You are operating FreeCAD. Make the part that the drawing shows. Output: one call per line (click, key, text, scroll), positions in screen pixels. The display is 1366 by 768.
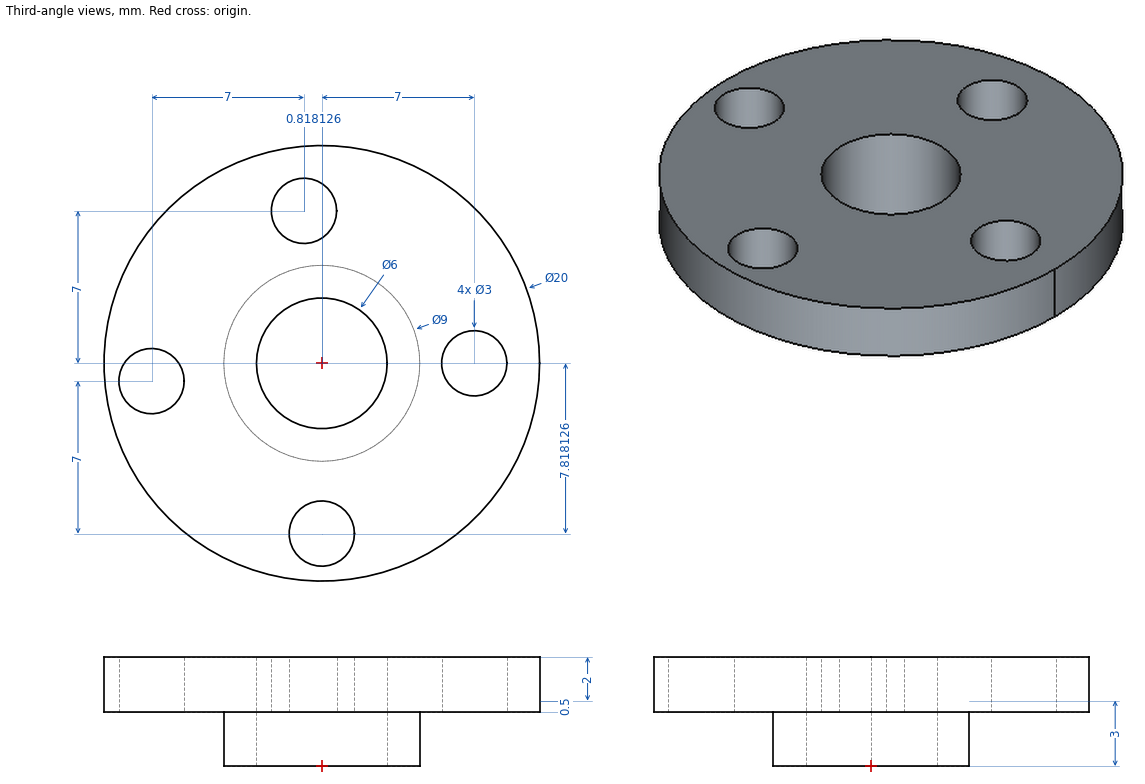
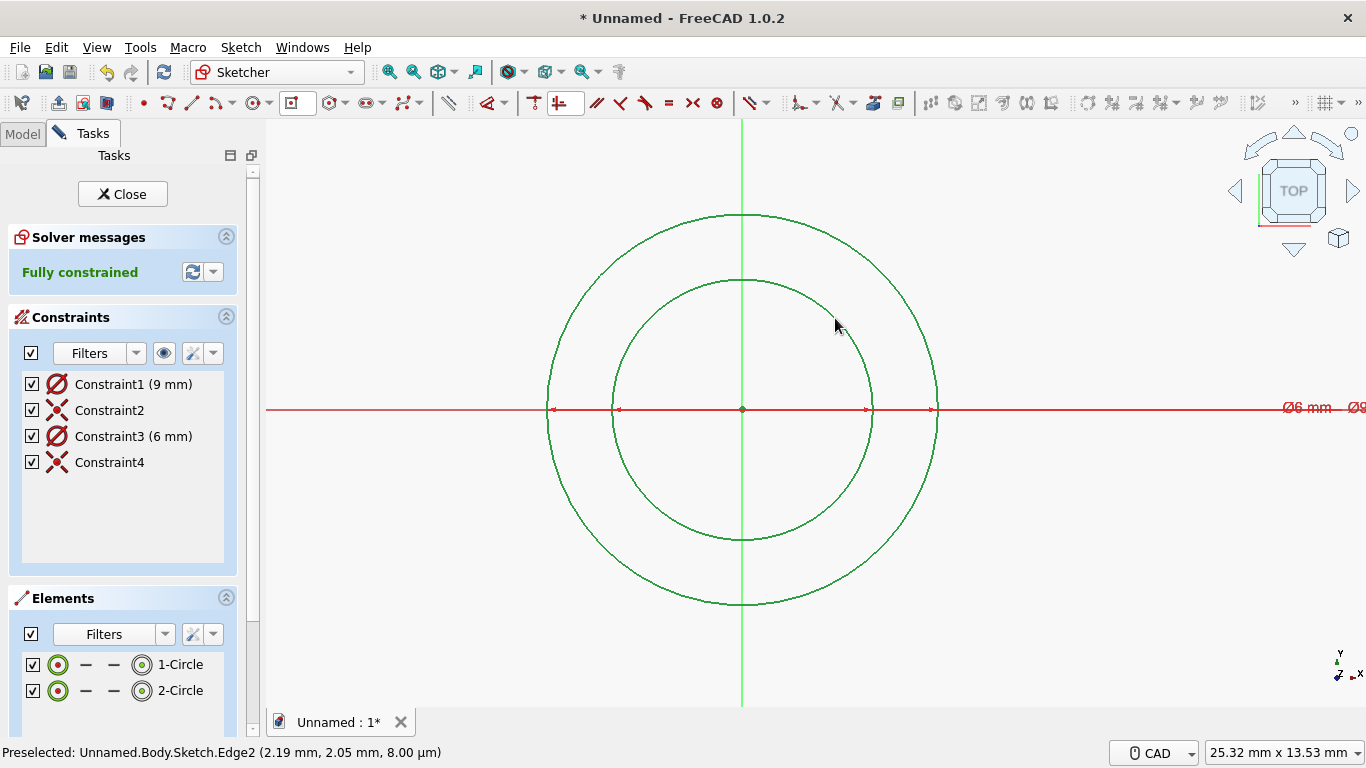
click(123, 194)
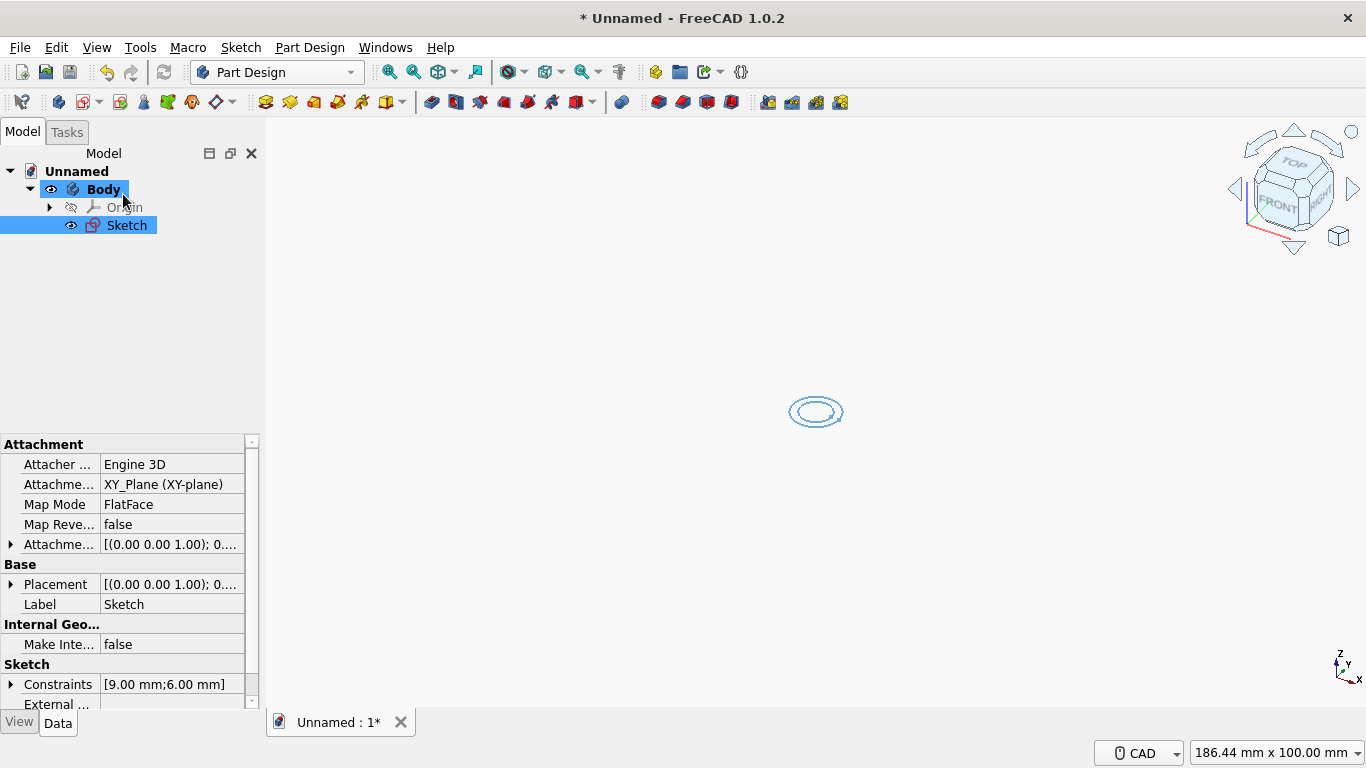
click(266, 102)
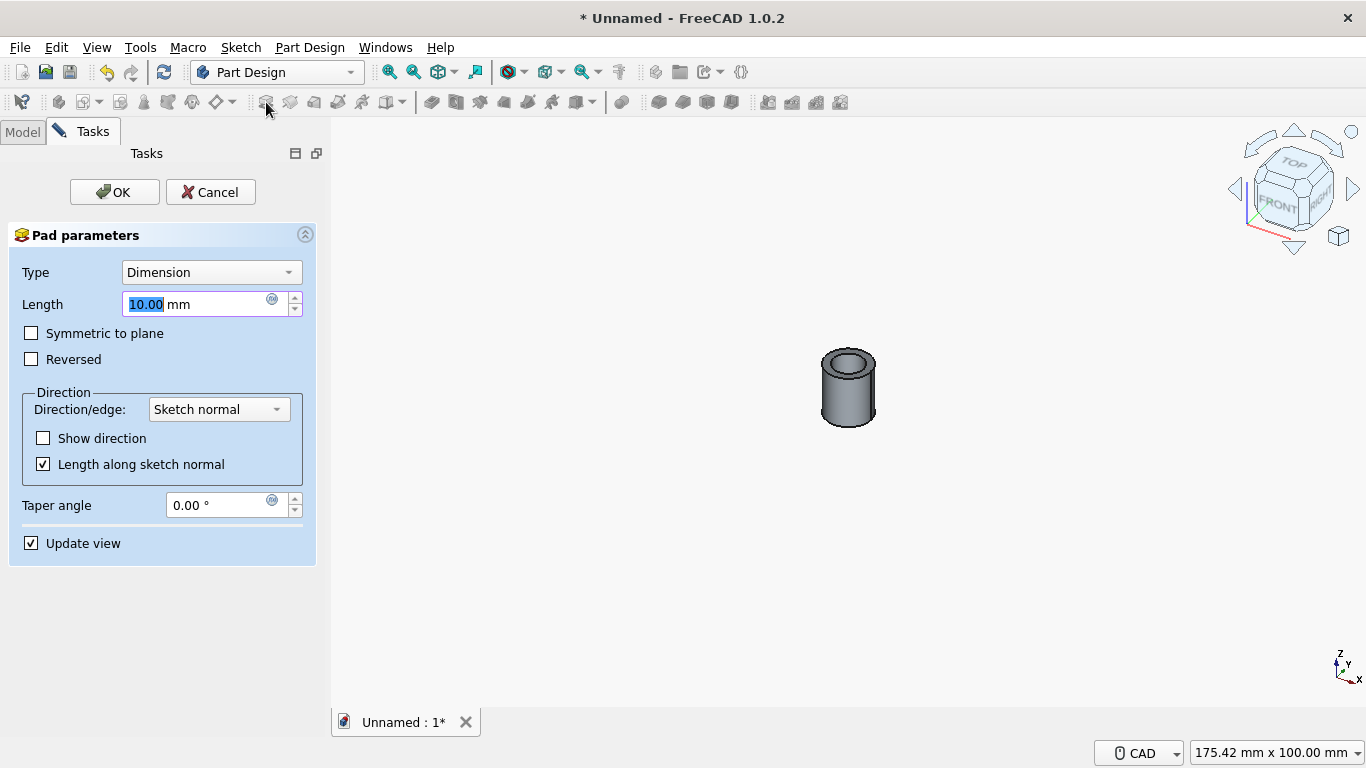
text(3)
key(Tab)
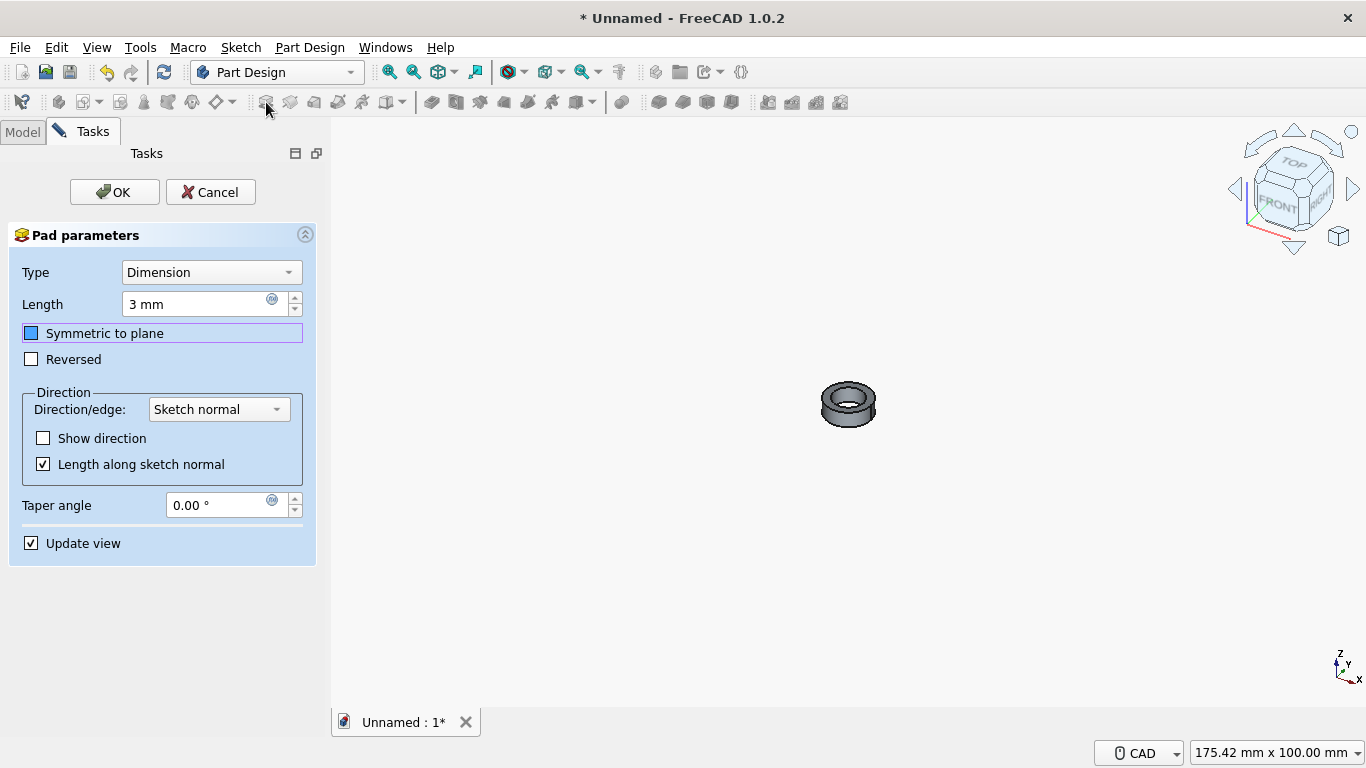
click(115, 192)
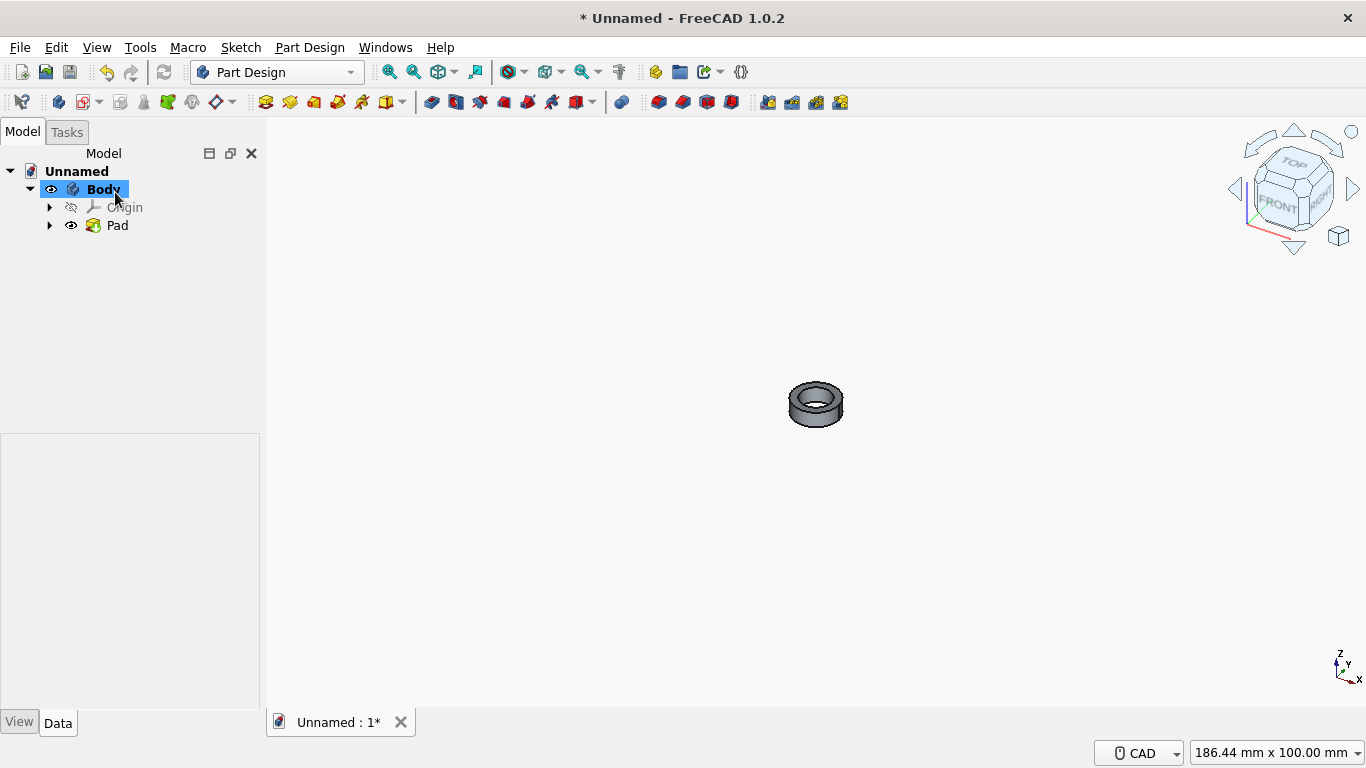
key(v)
key(f)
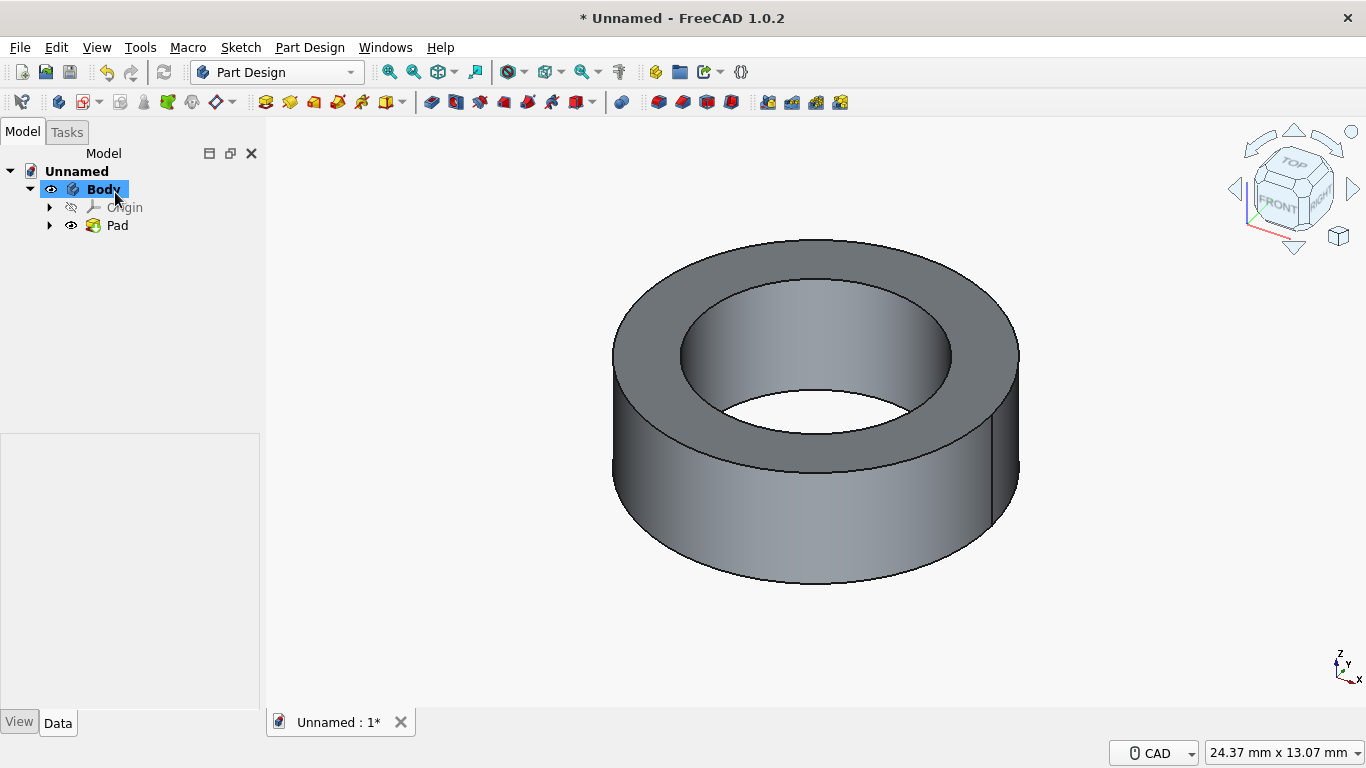
click(729, 442)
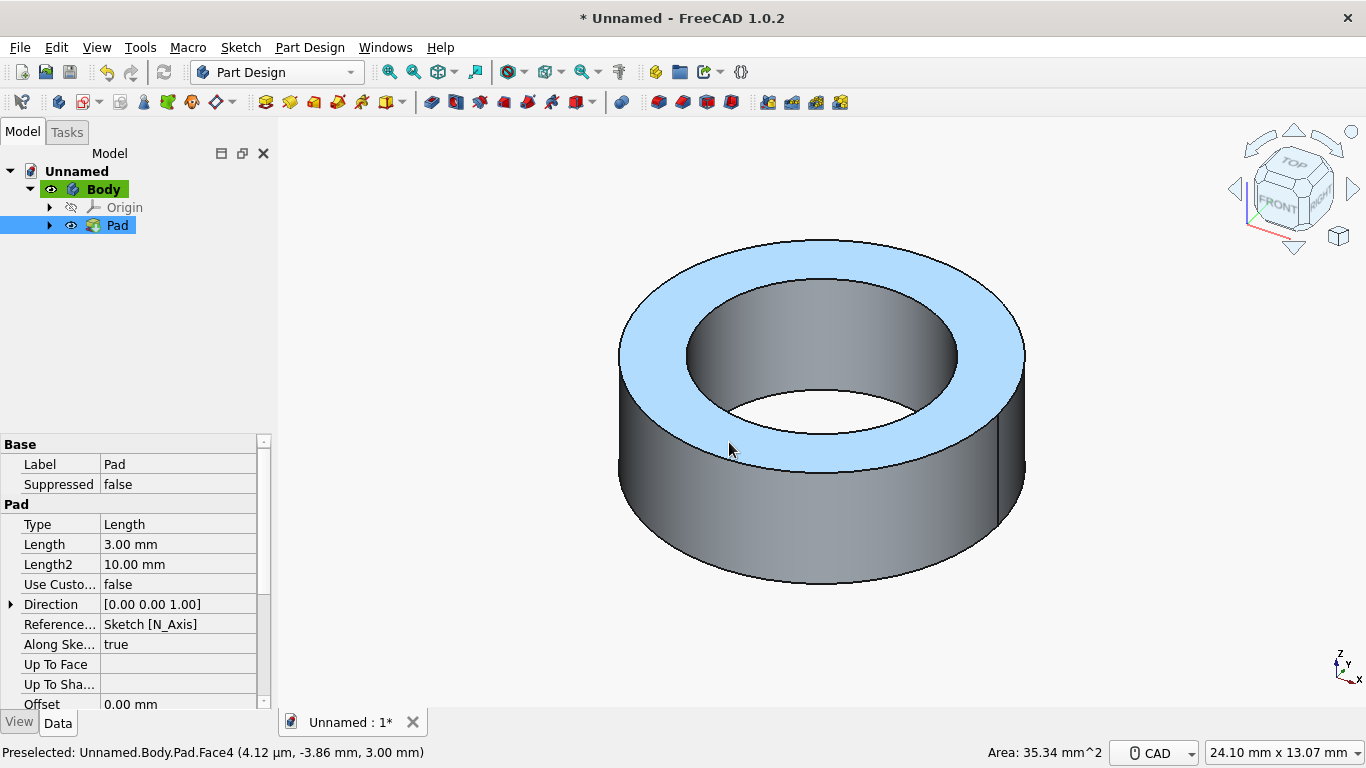
click(84, 102)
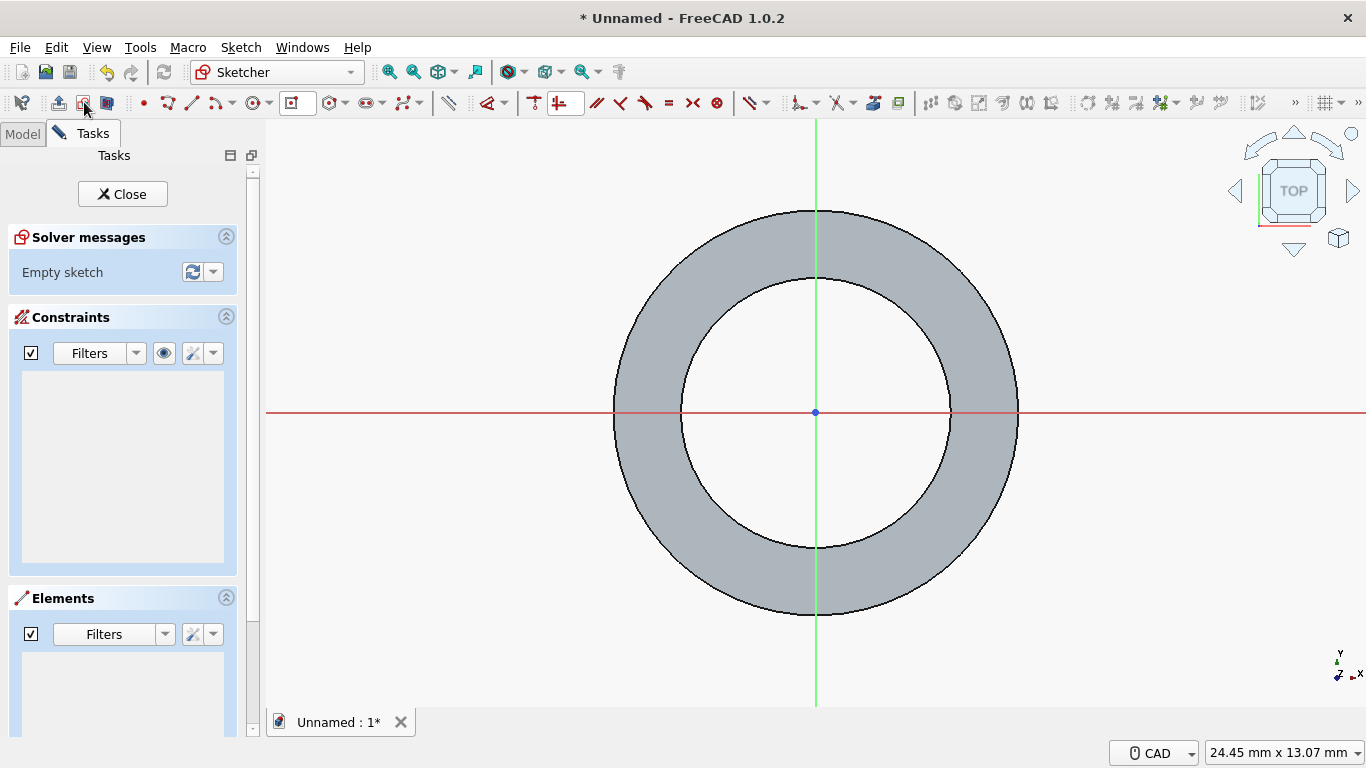
scroll(692, 413, down, 4)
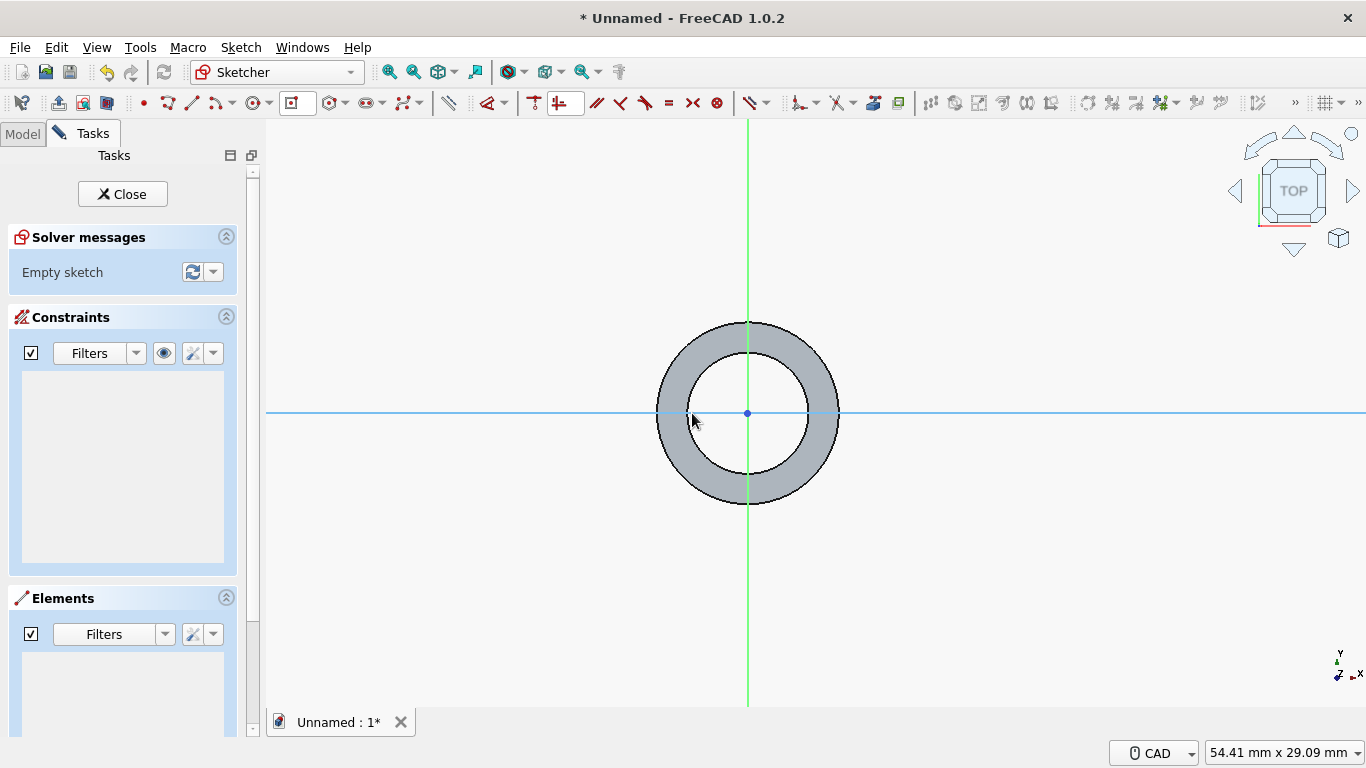
click(254, 104)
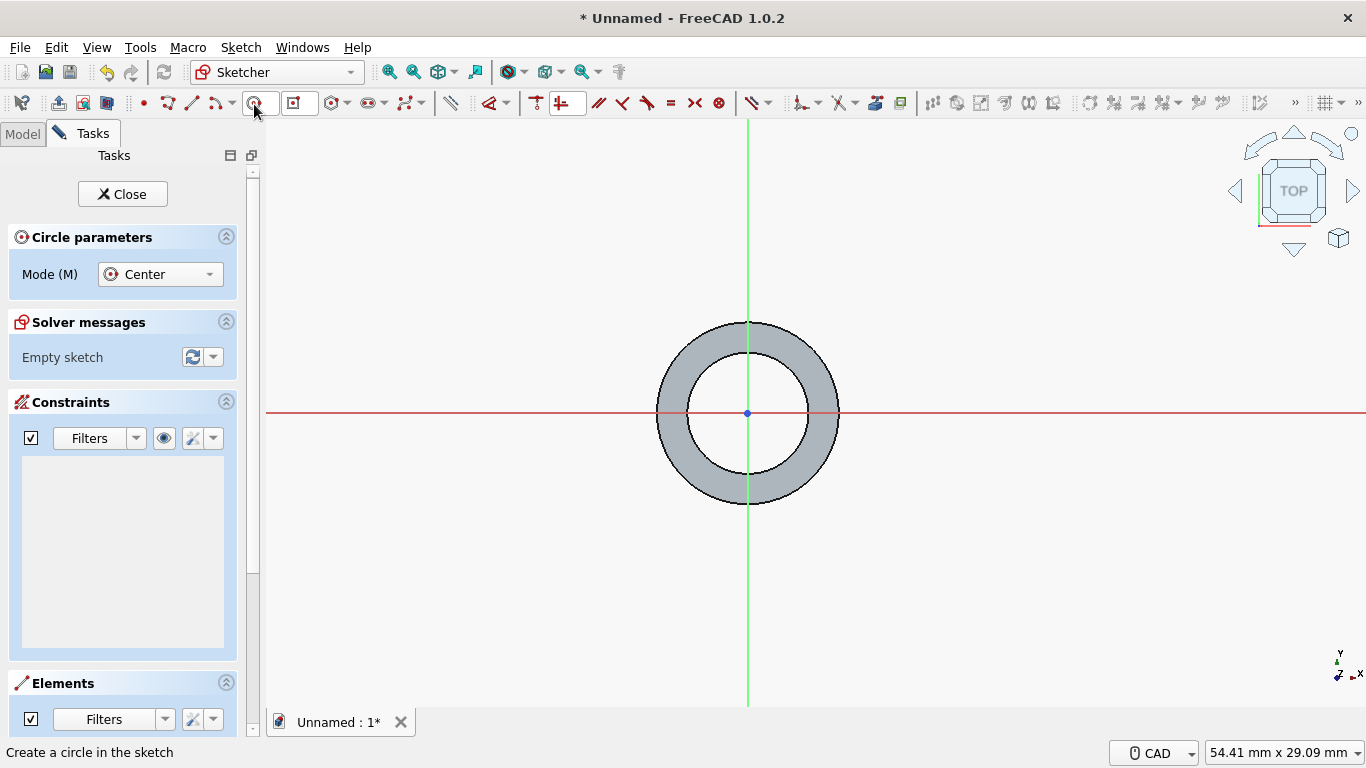
click(748, 413)
move(891, 270)